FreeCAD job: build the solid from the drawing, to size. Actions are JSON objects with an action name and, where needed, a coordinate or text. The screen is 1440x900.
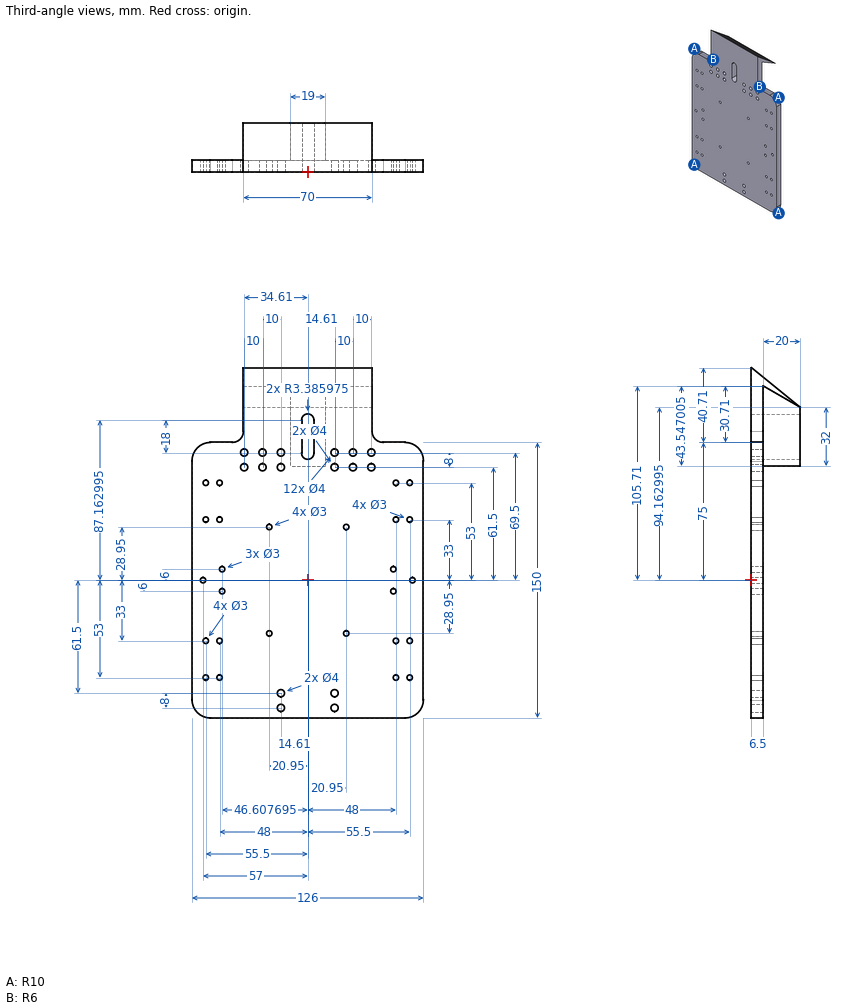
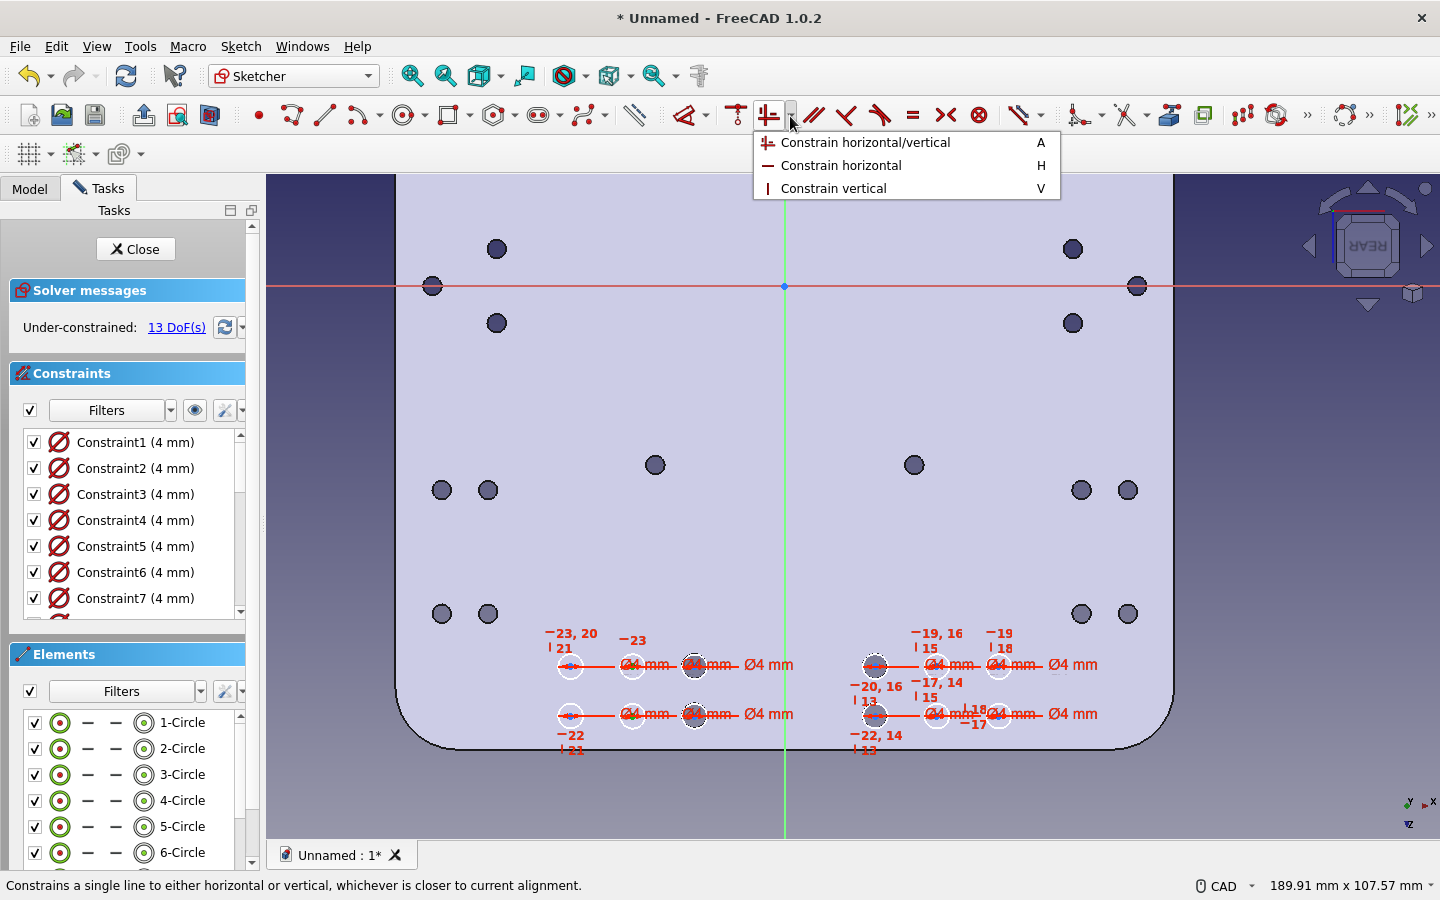
{"action": "left_click", "coordinate": [907, 188]}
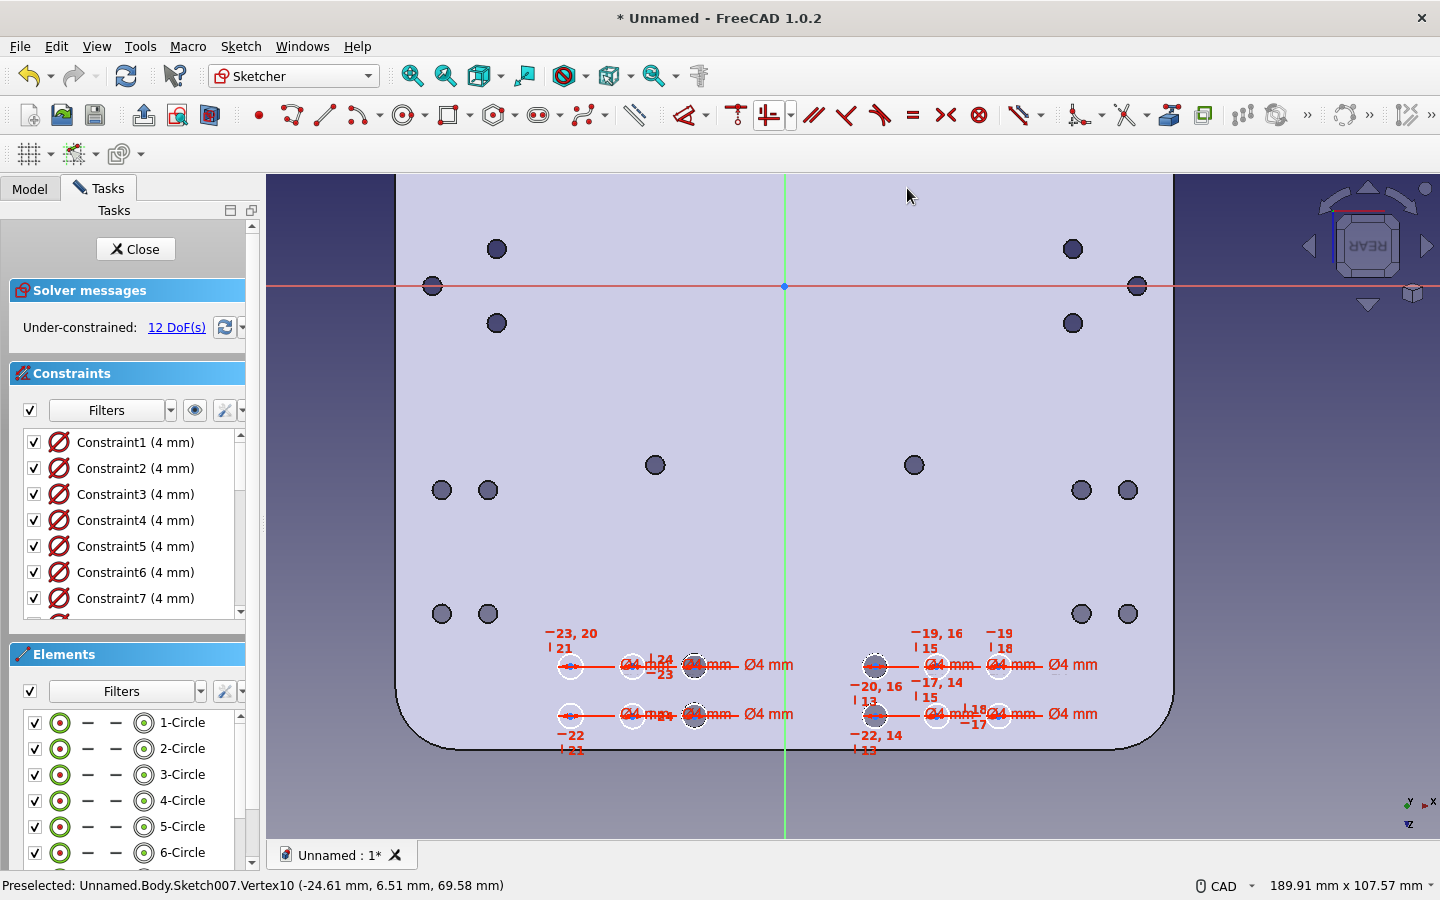
{"action": "left_click", "coordinate": [571, 716]}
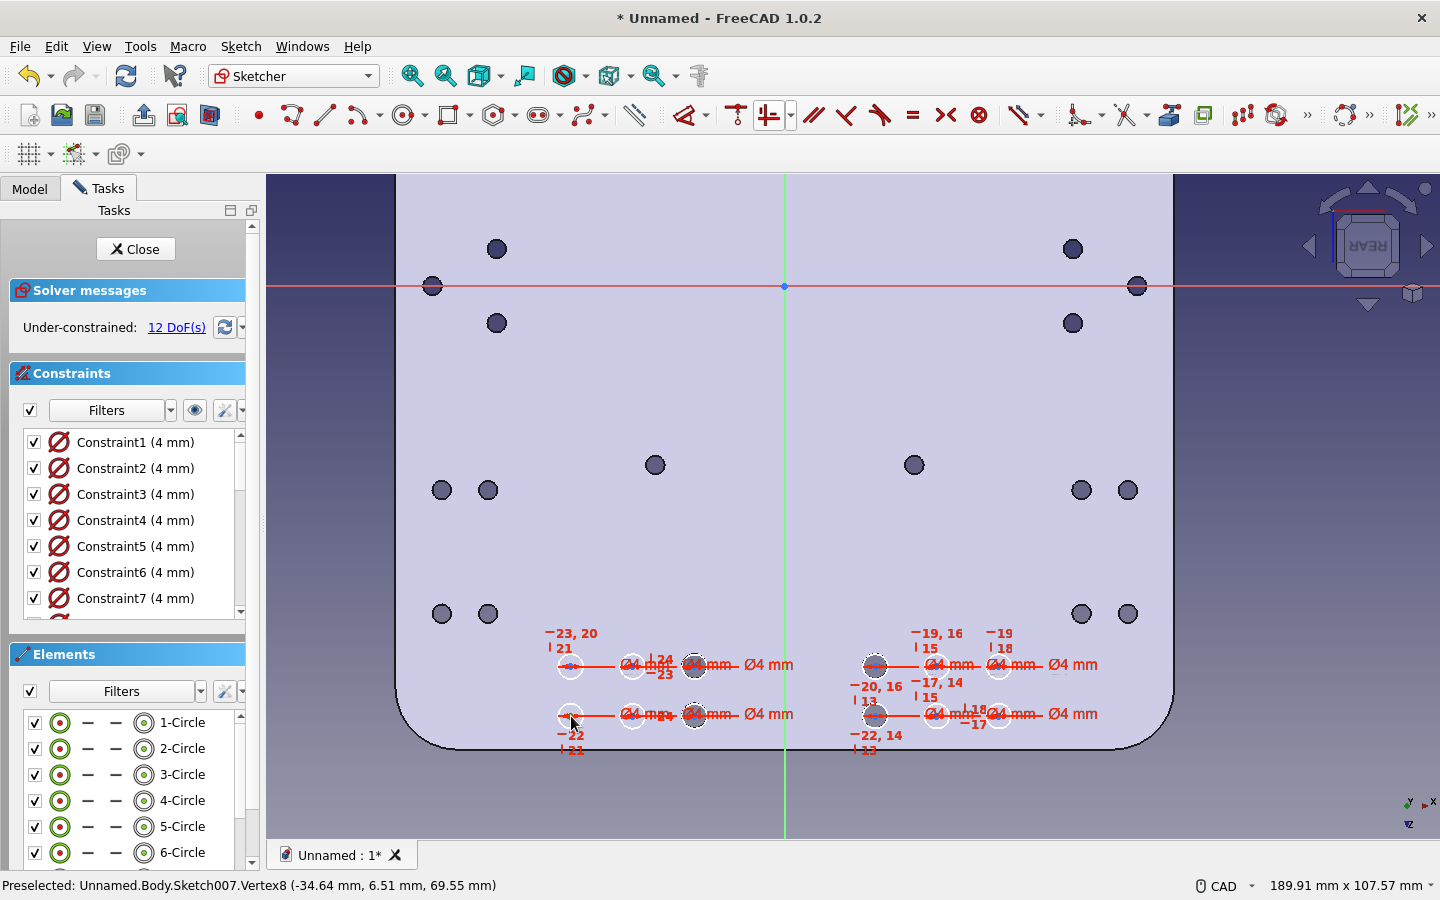
{"action": "left_click", "coordinate": [633, 716]}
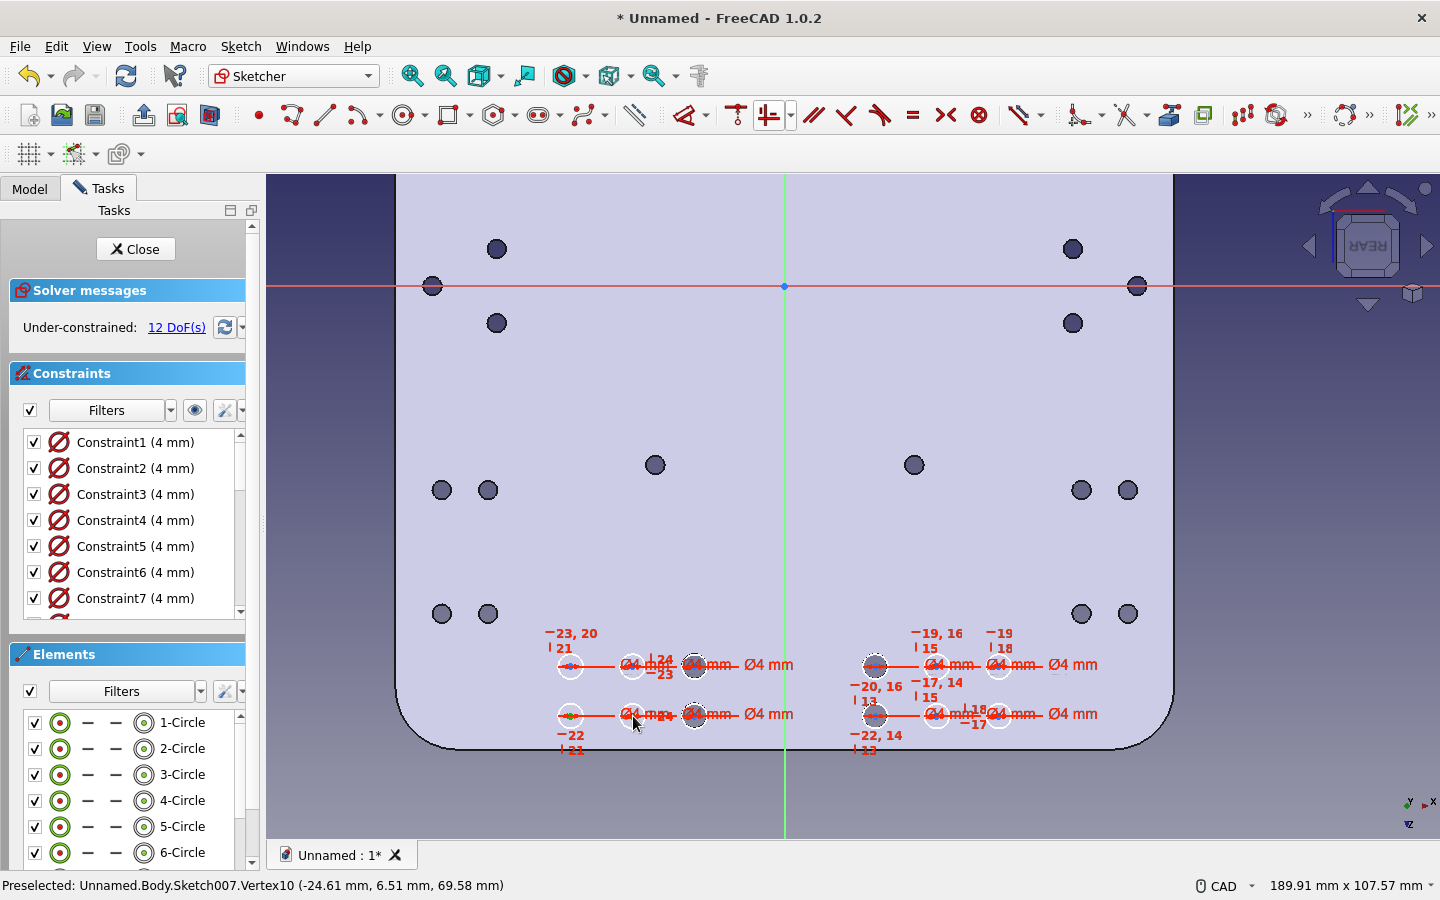
{"action": "key", "text": "h"}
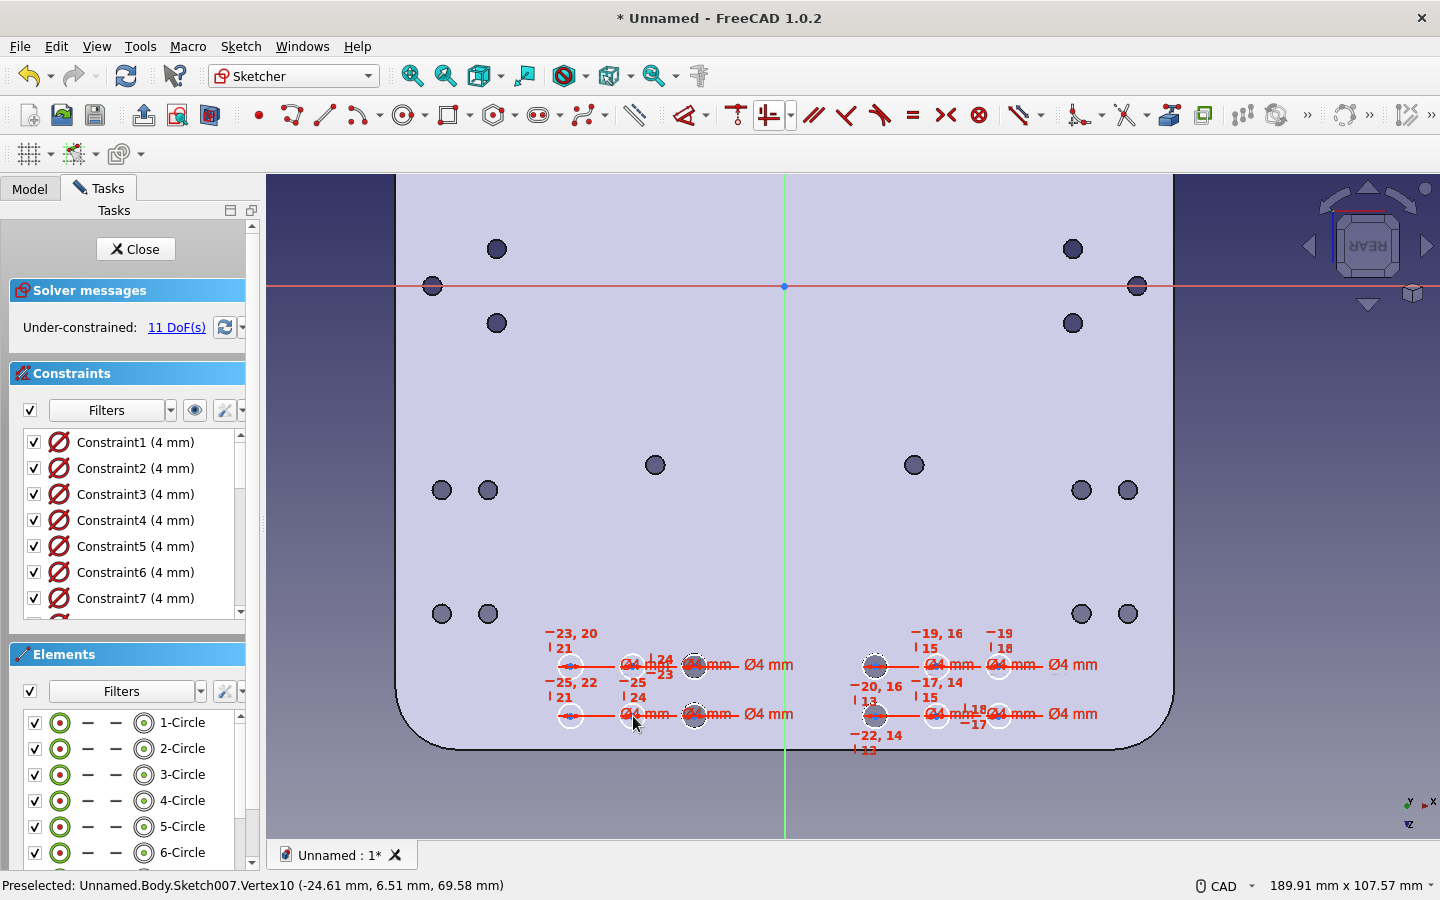
{"action": "left_click", "coordinate": [633, 667]}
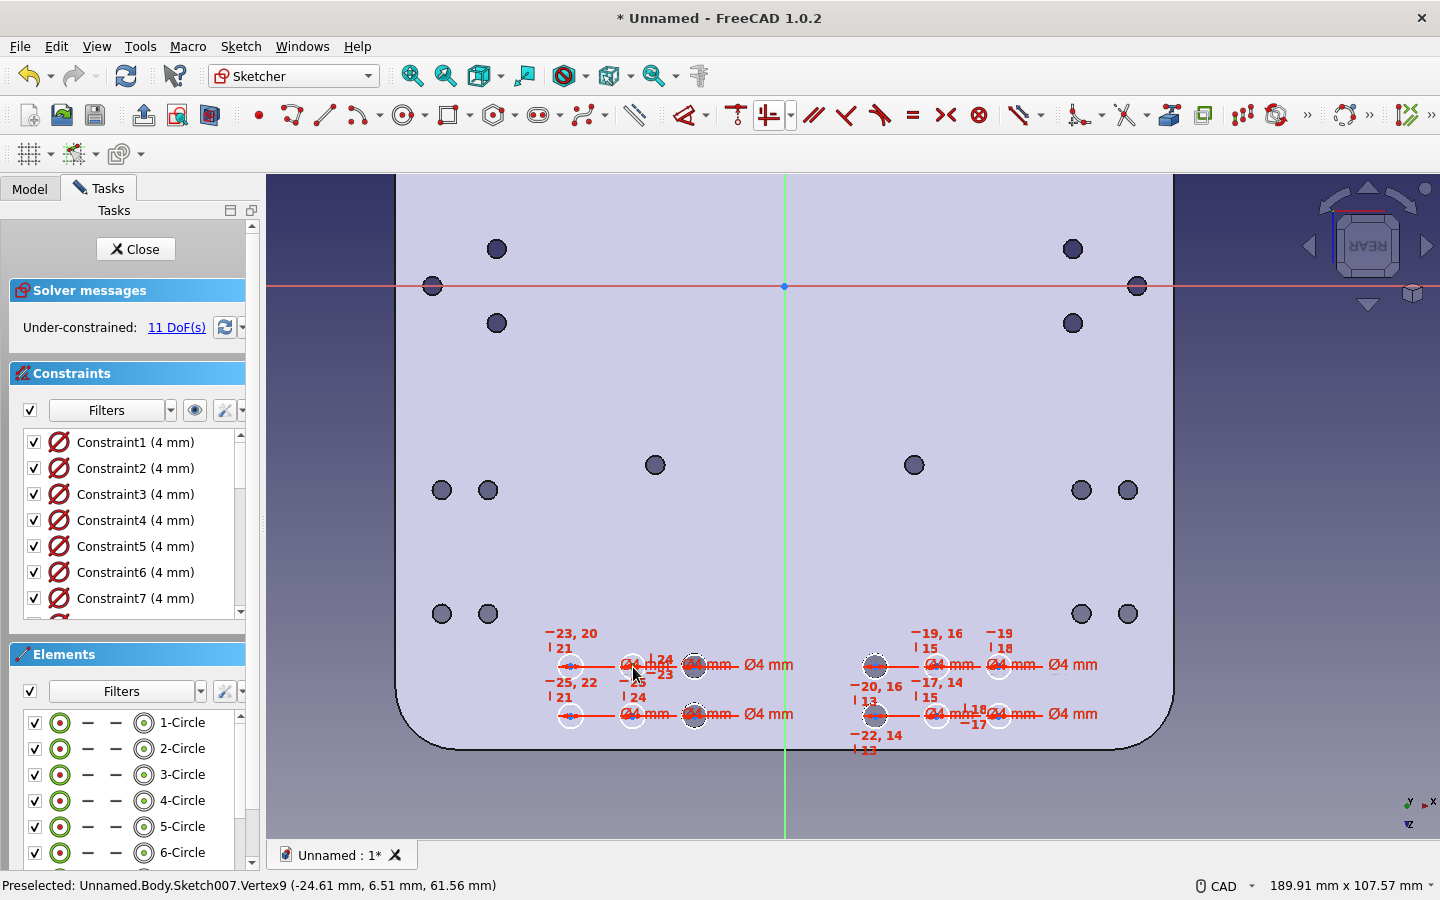
{"action": "left_click", "coordinate": [695, 667]}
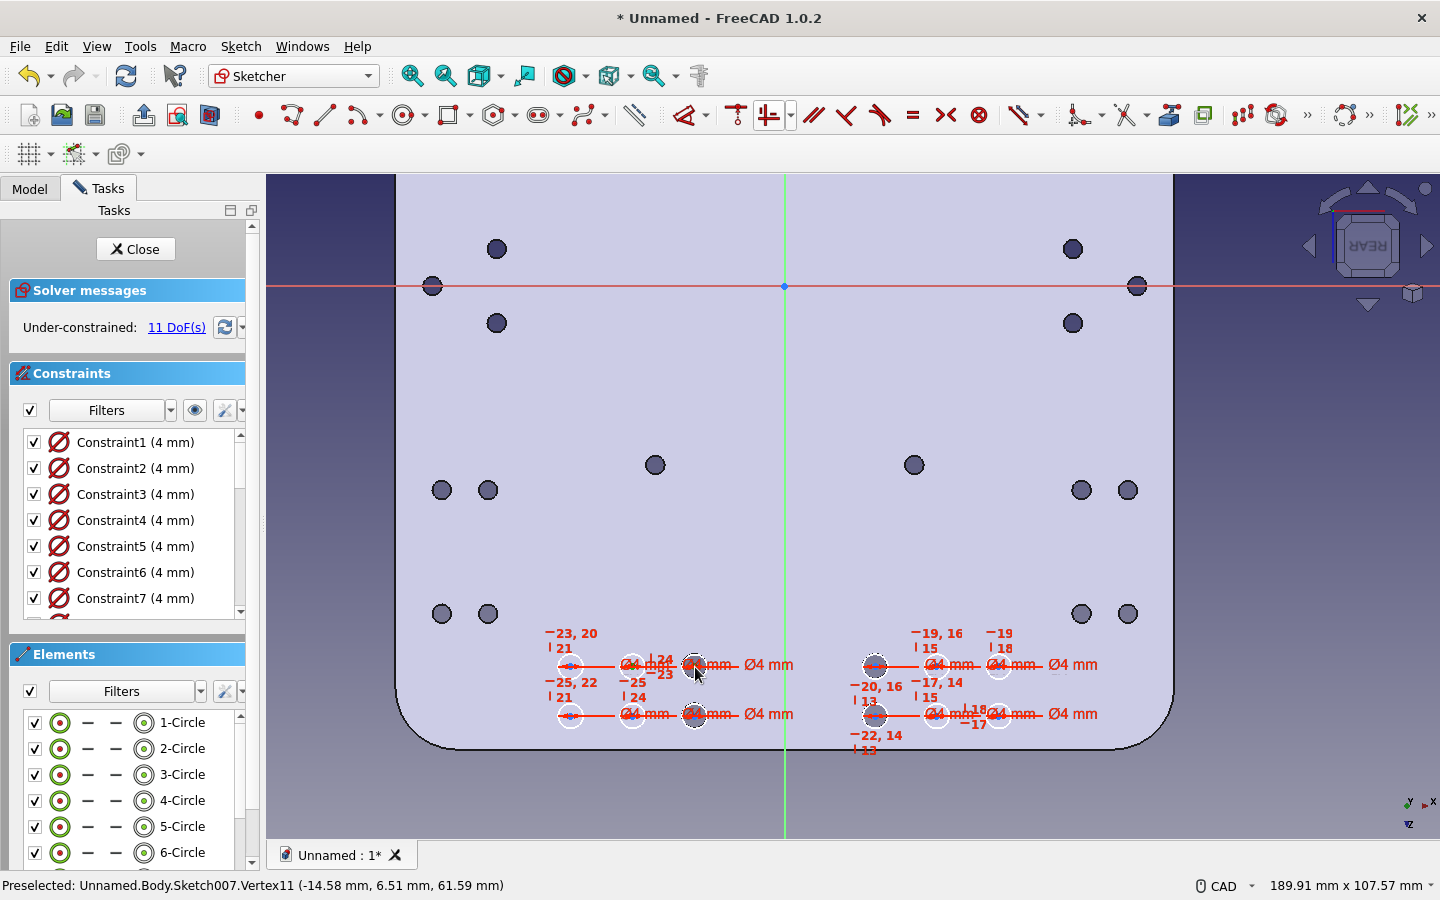
{"action": "left_click", "coordinate": [790, 116]}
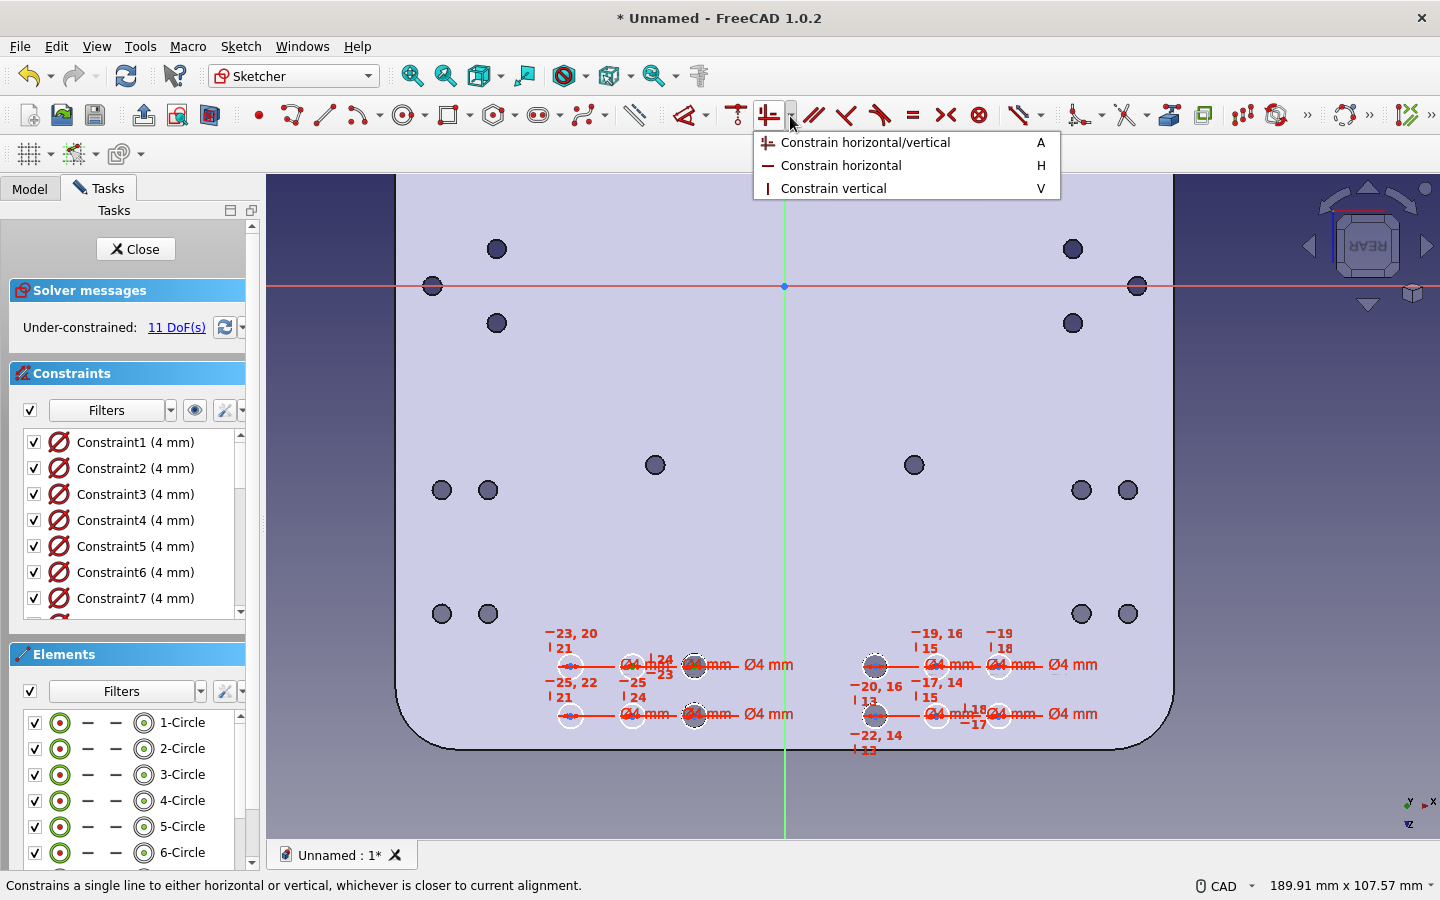
{"action": "left_click", "coordinate": [907, 166]}